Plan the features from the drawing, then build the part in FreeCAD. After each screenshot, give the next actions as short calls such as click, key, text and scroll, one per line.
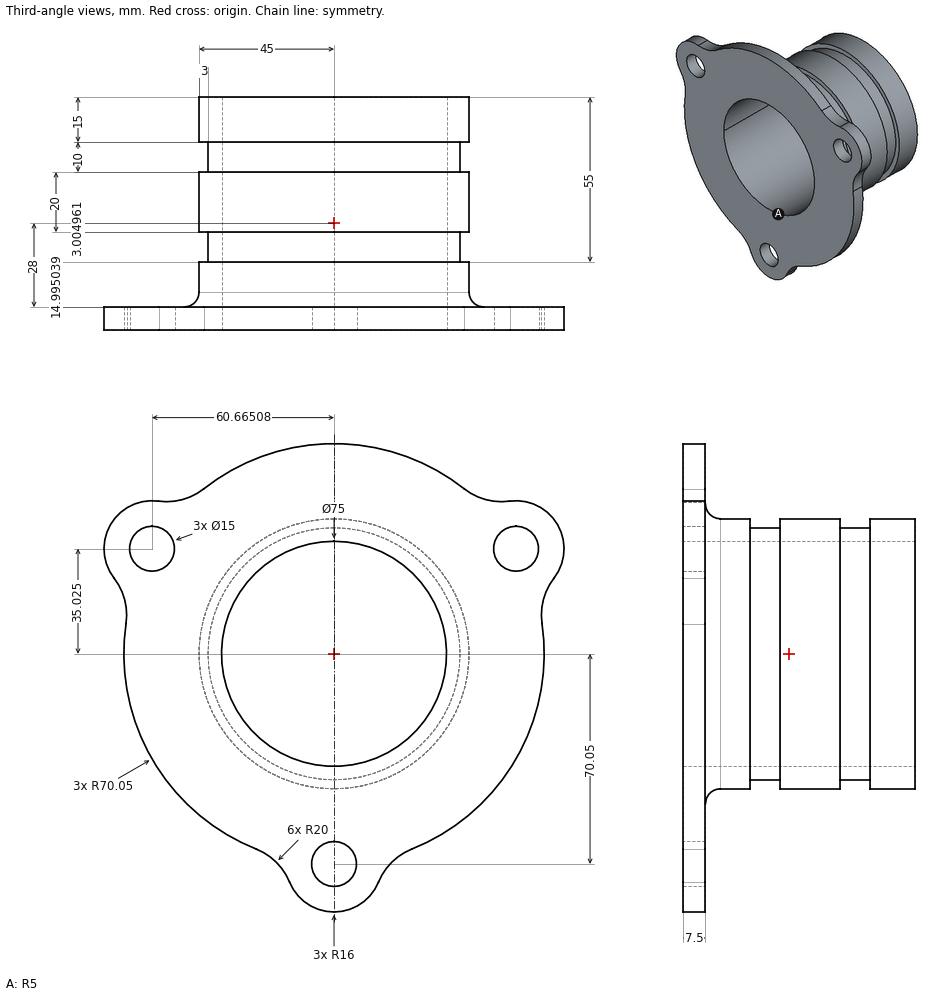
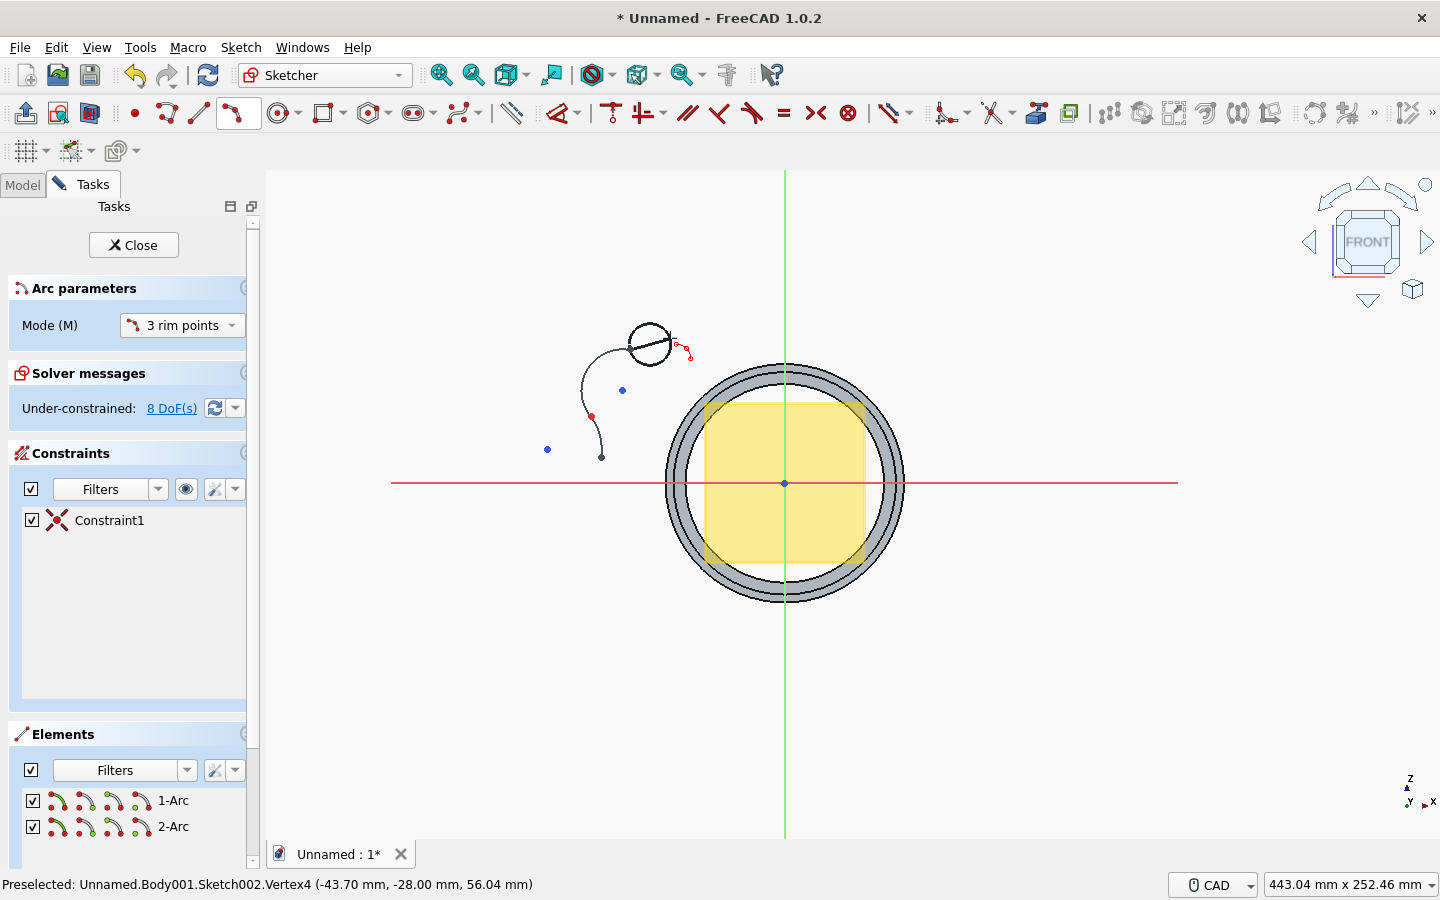
scroll(651, 347, up, 7)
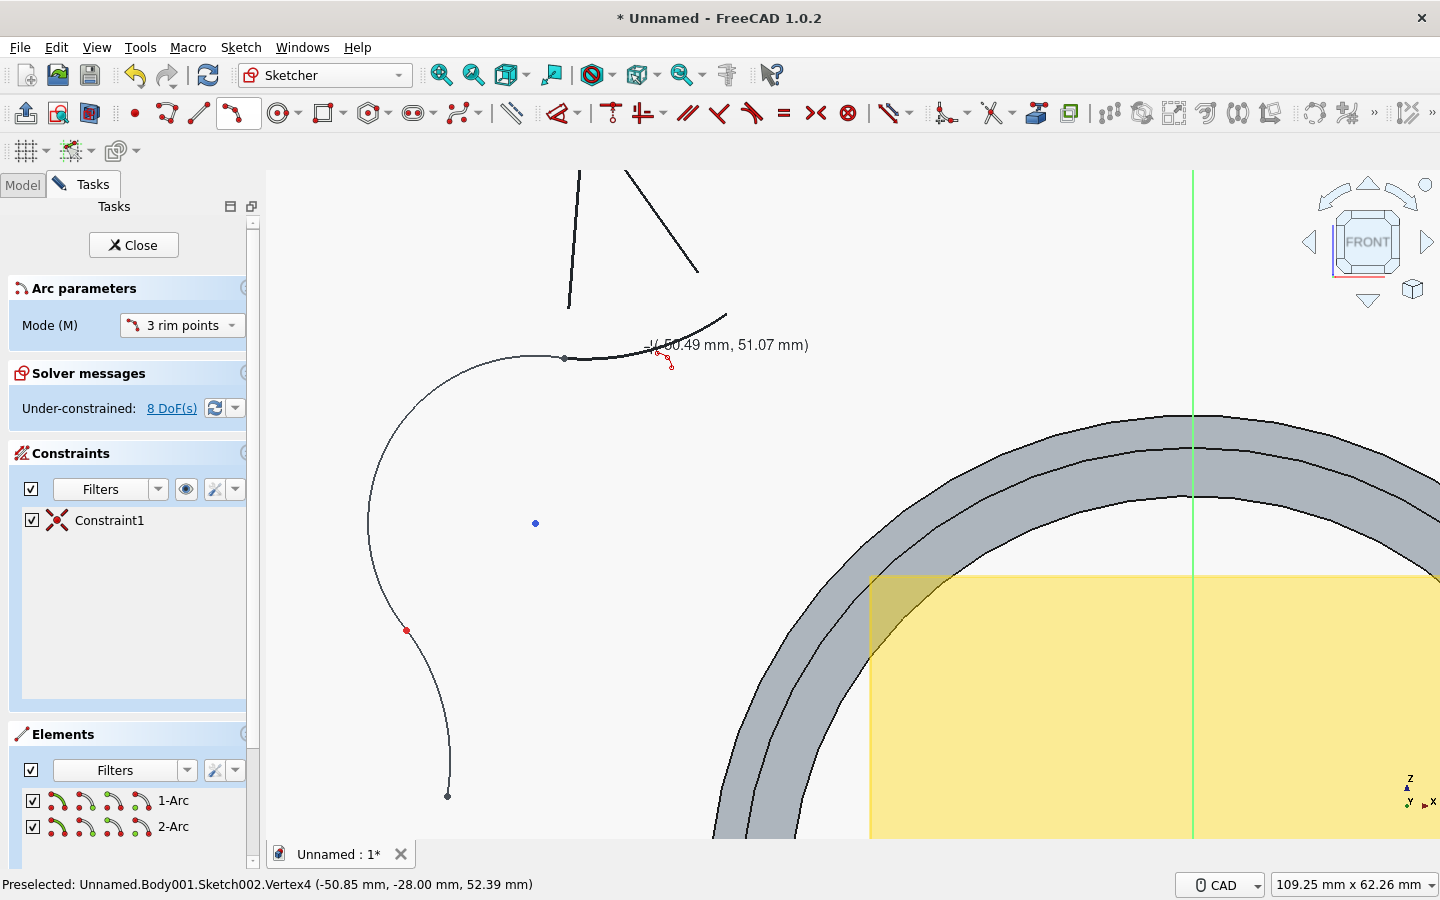
click(650, 347)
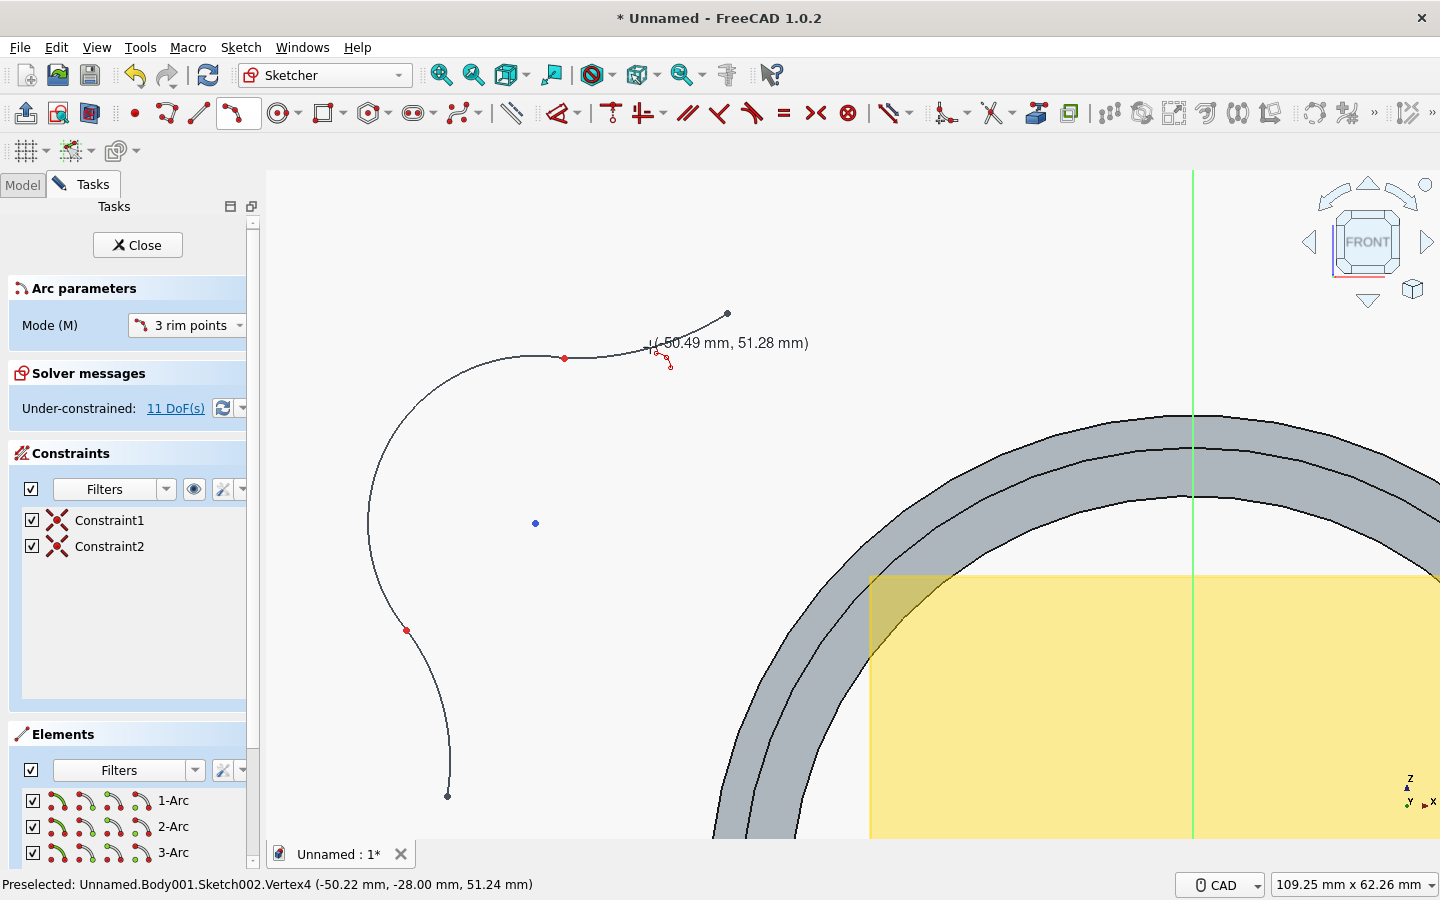
scroll(651, 347, down, 7)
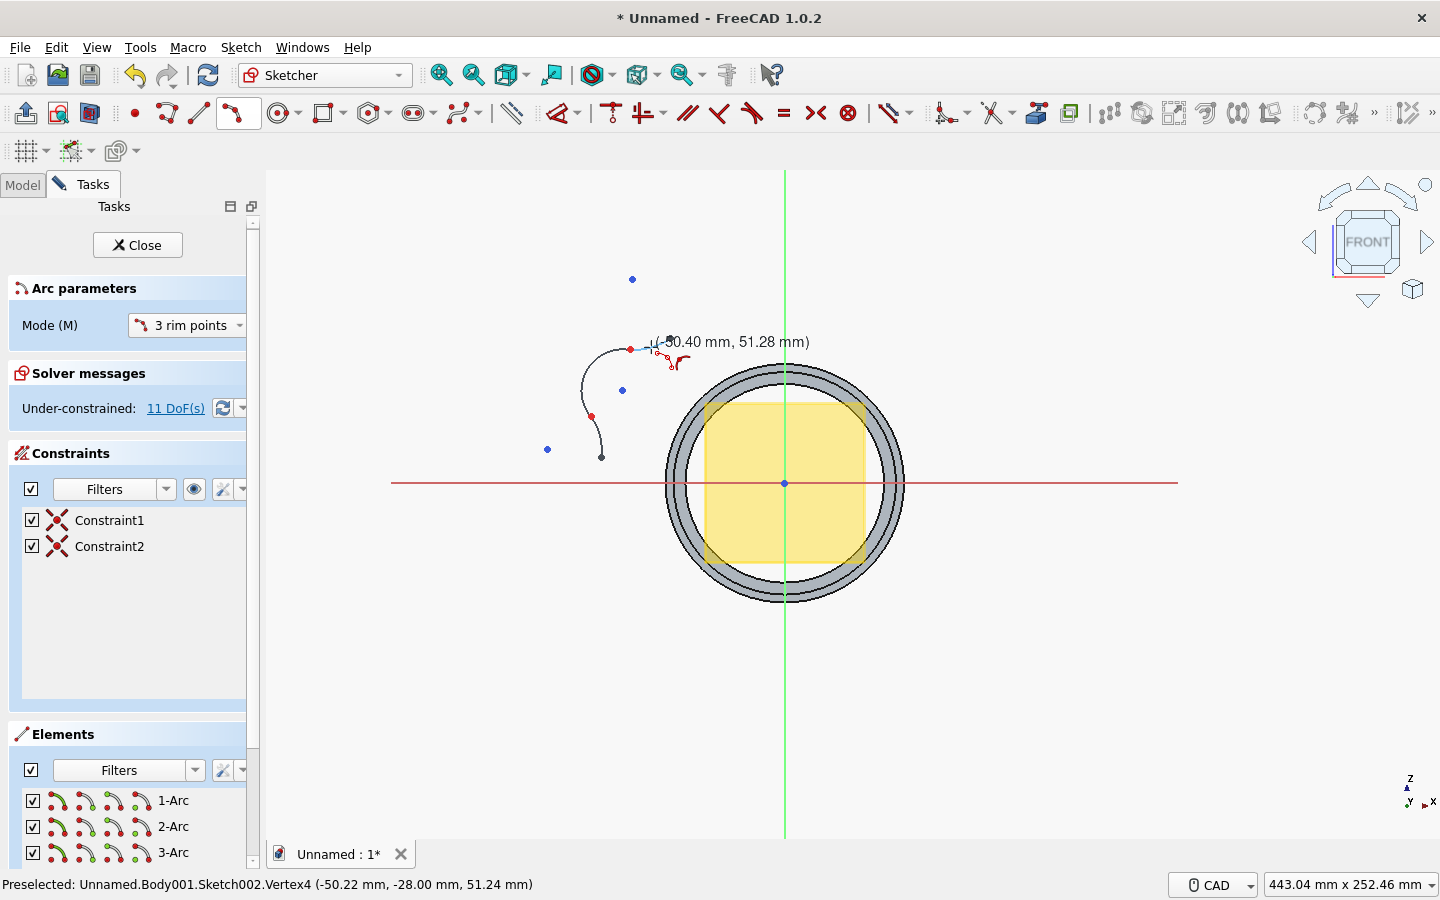
click(670, 339)
click(900, 338)
click(810, 299)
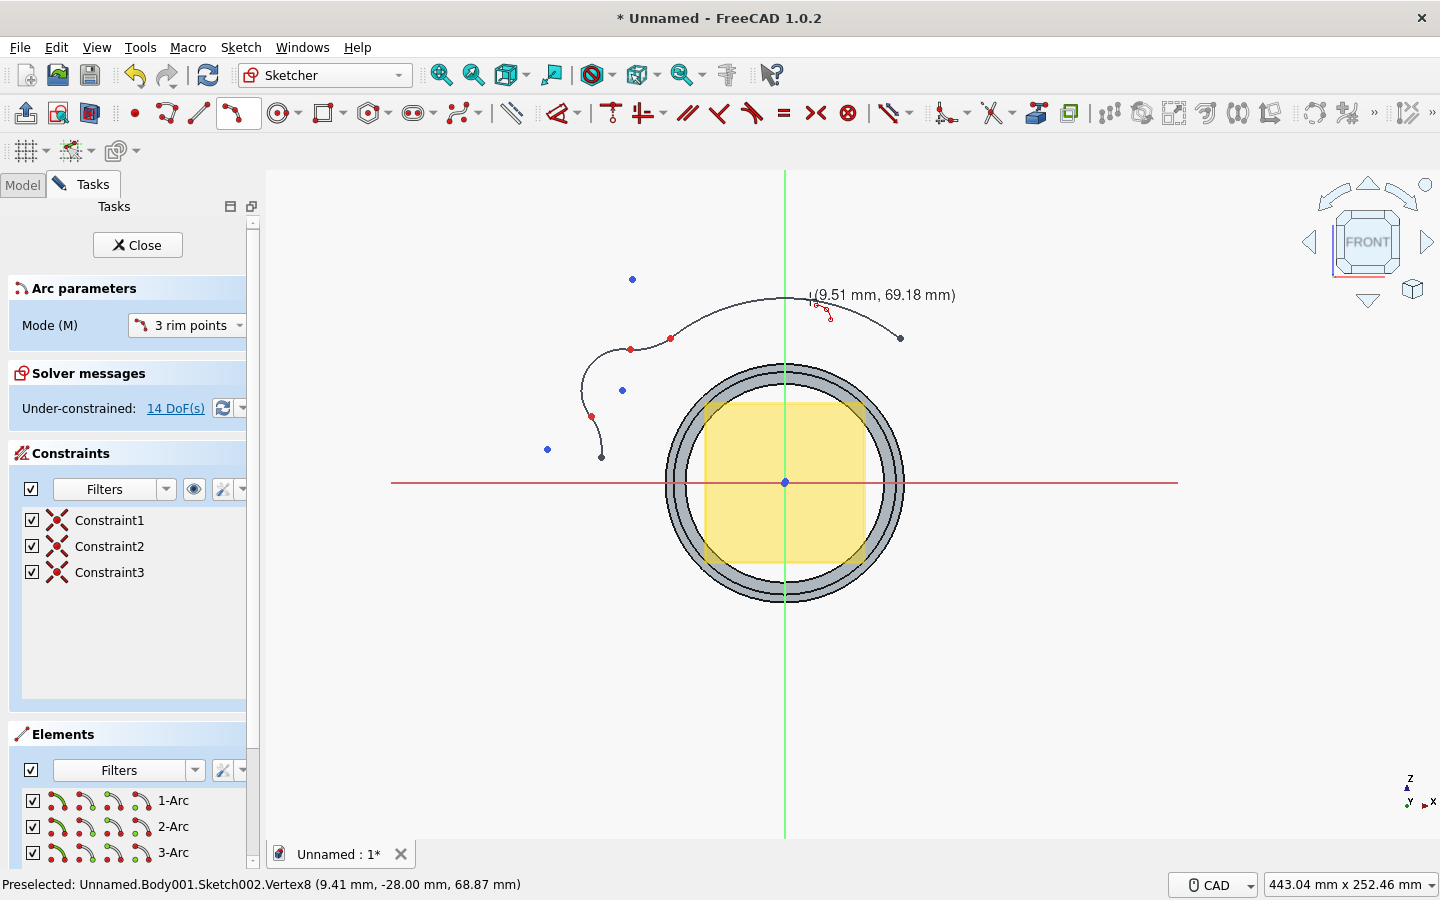
click(900, 339)
click(940, 349)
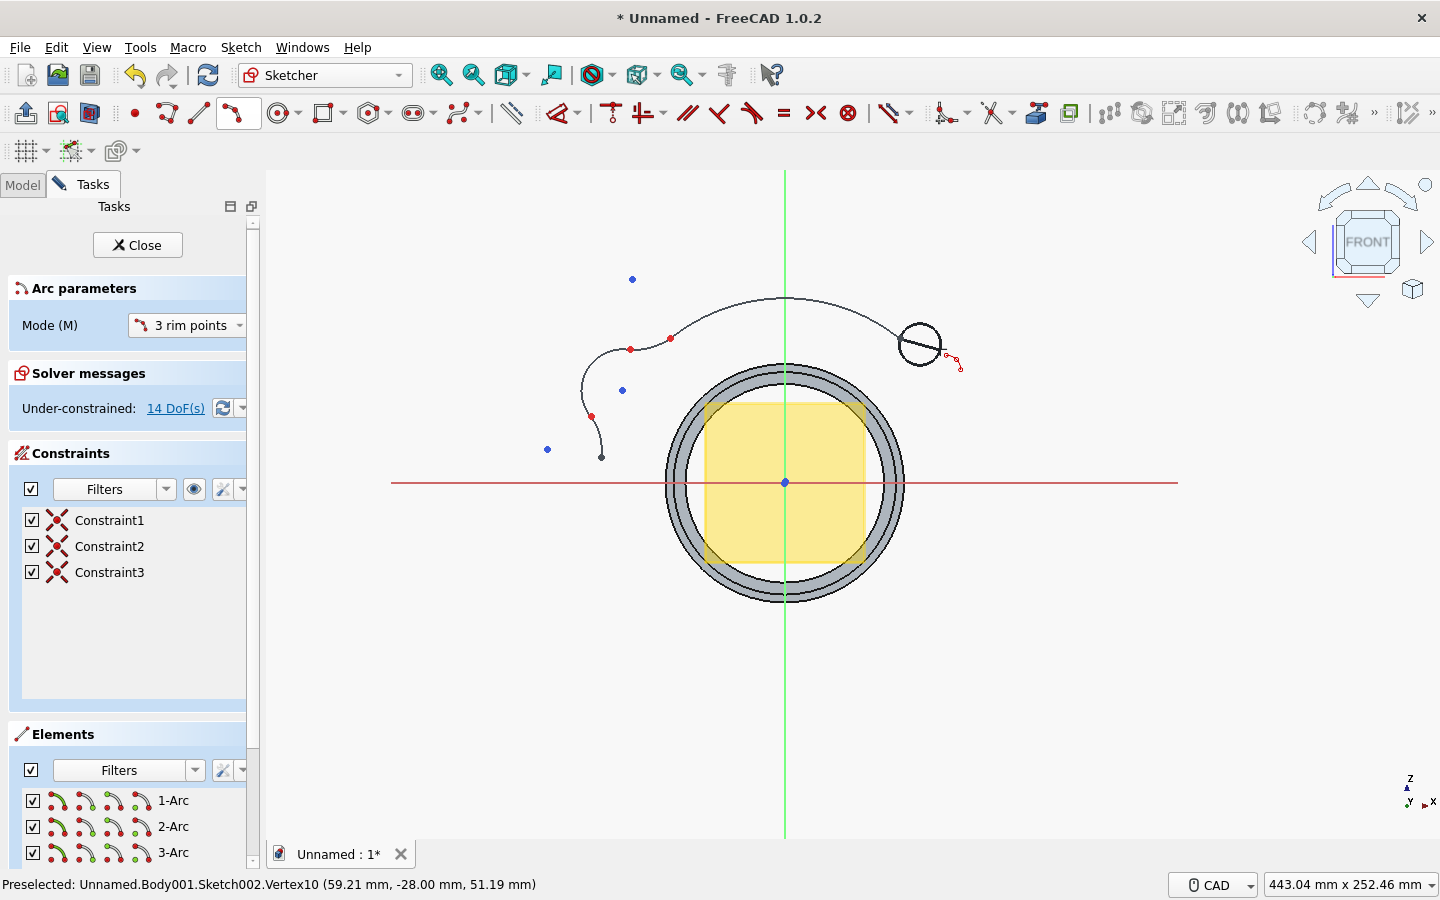
scroll(919, 347, up, 7)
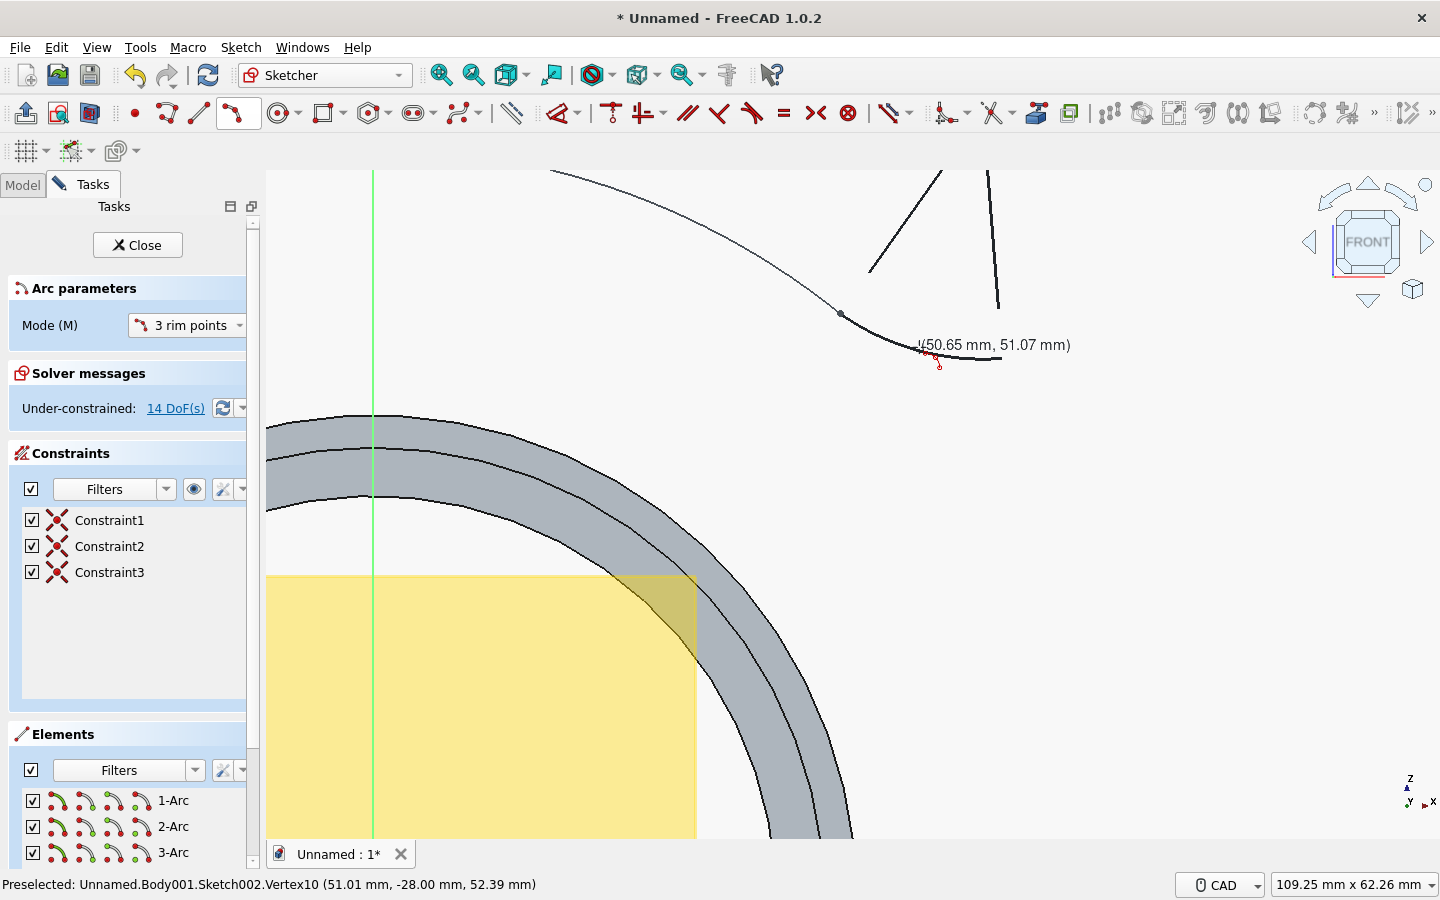
click(916, 347)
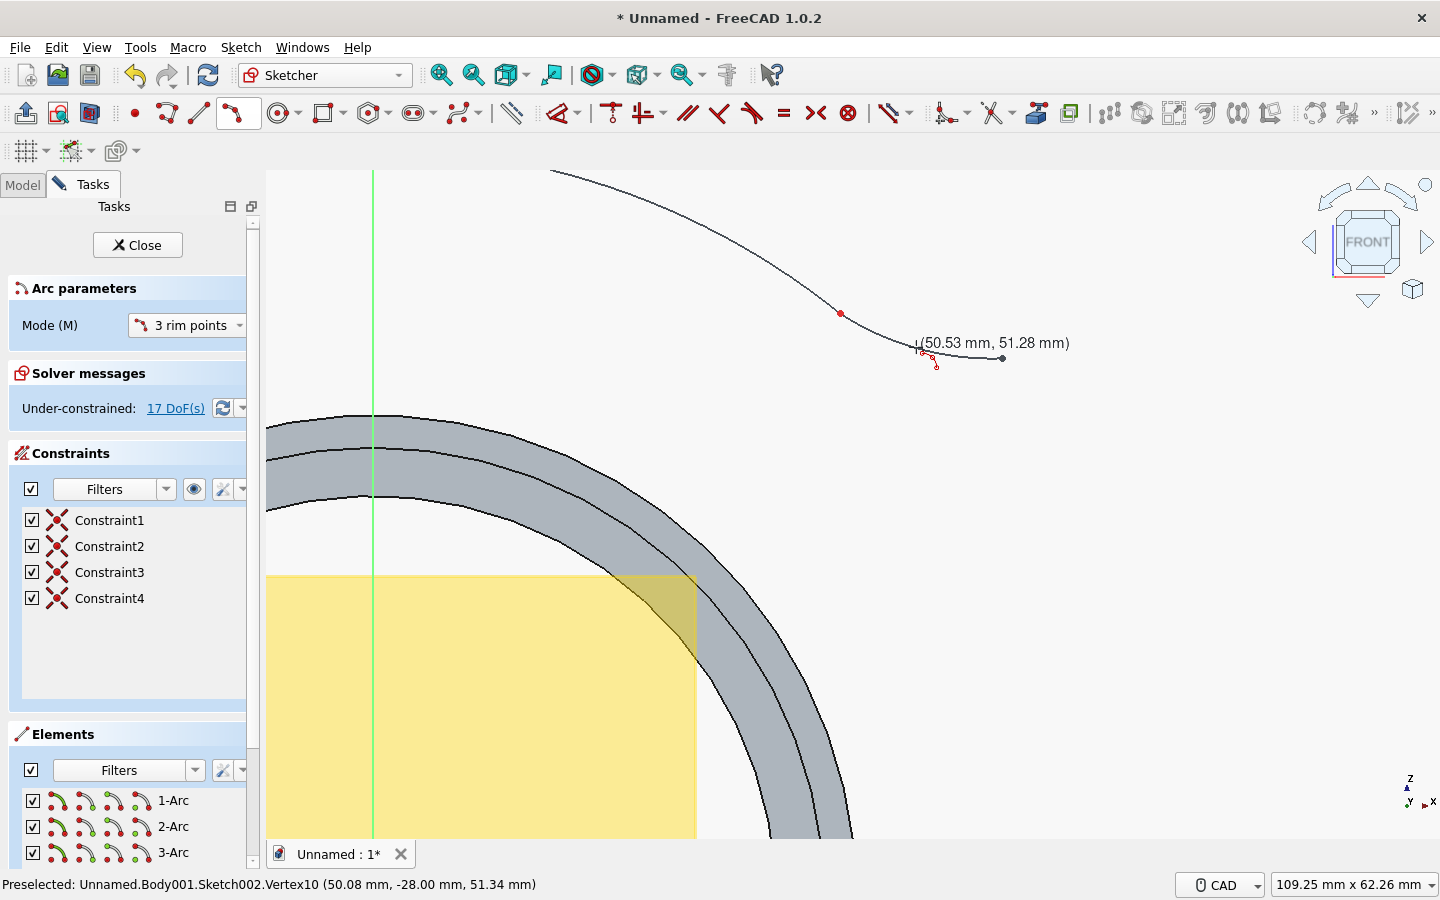
scroll(919, 347, down, 7)